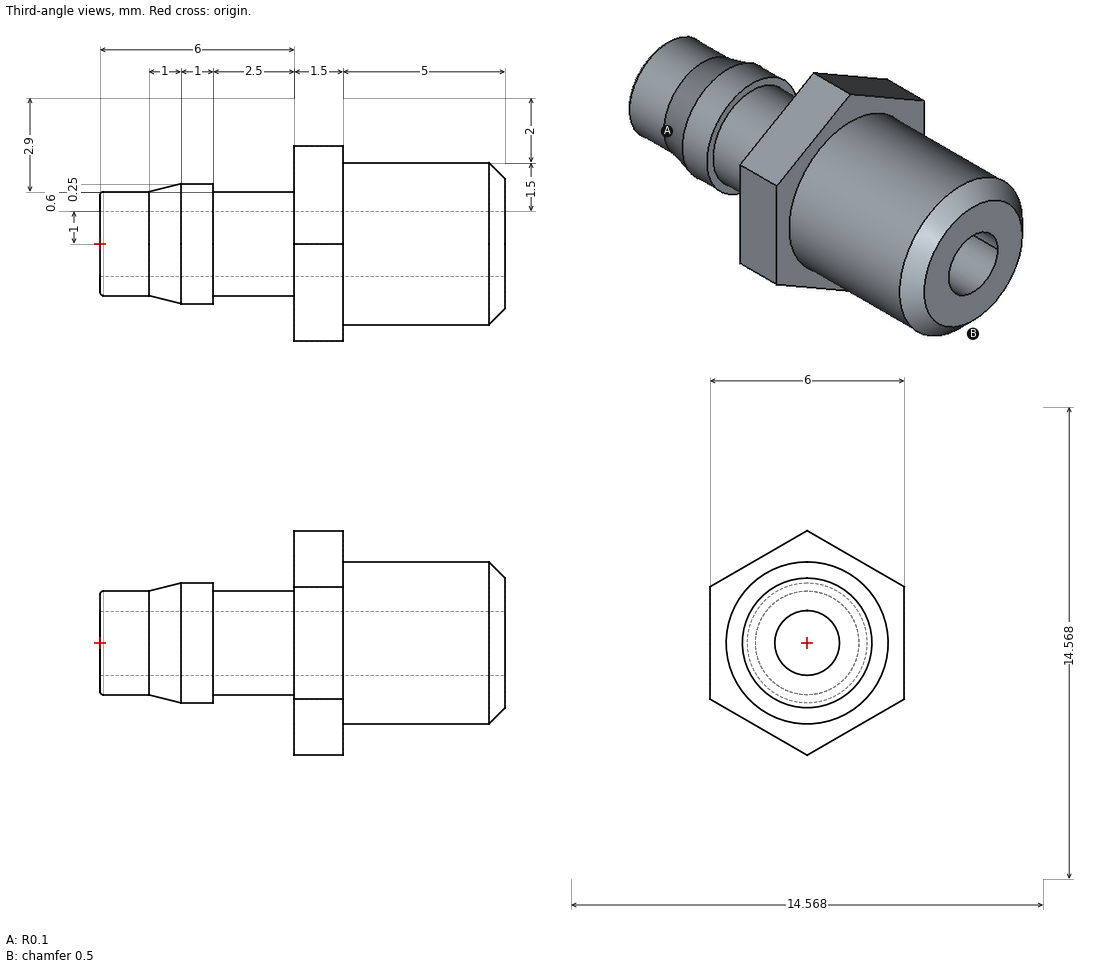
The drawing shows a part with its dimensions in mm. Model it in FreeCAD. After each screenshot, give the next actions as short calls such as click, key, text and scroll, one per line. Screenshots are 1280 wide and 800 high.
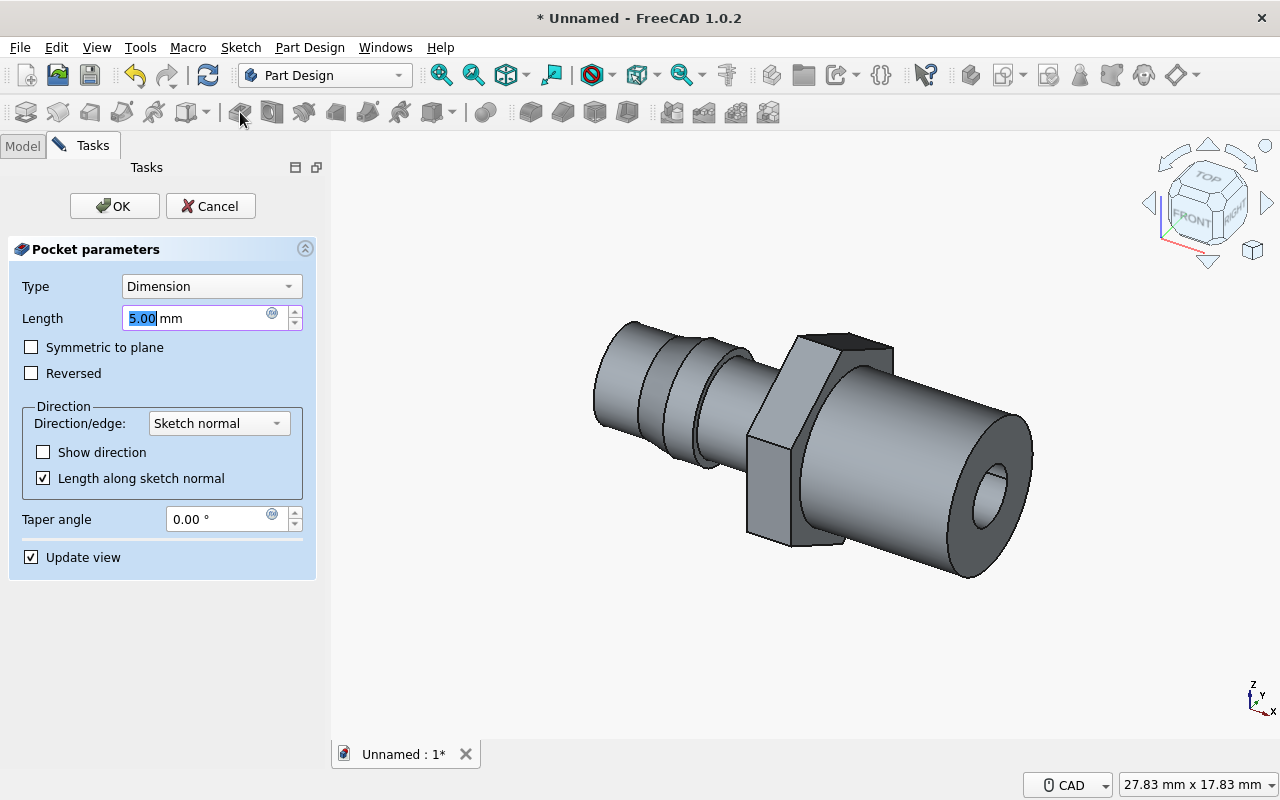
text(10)
key(Tab)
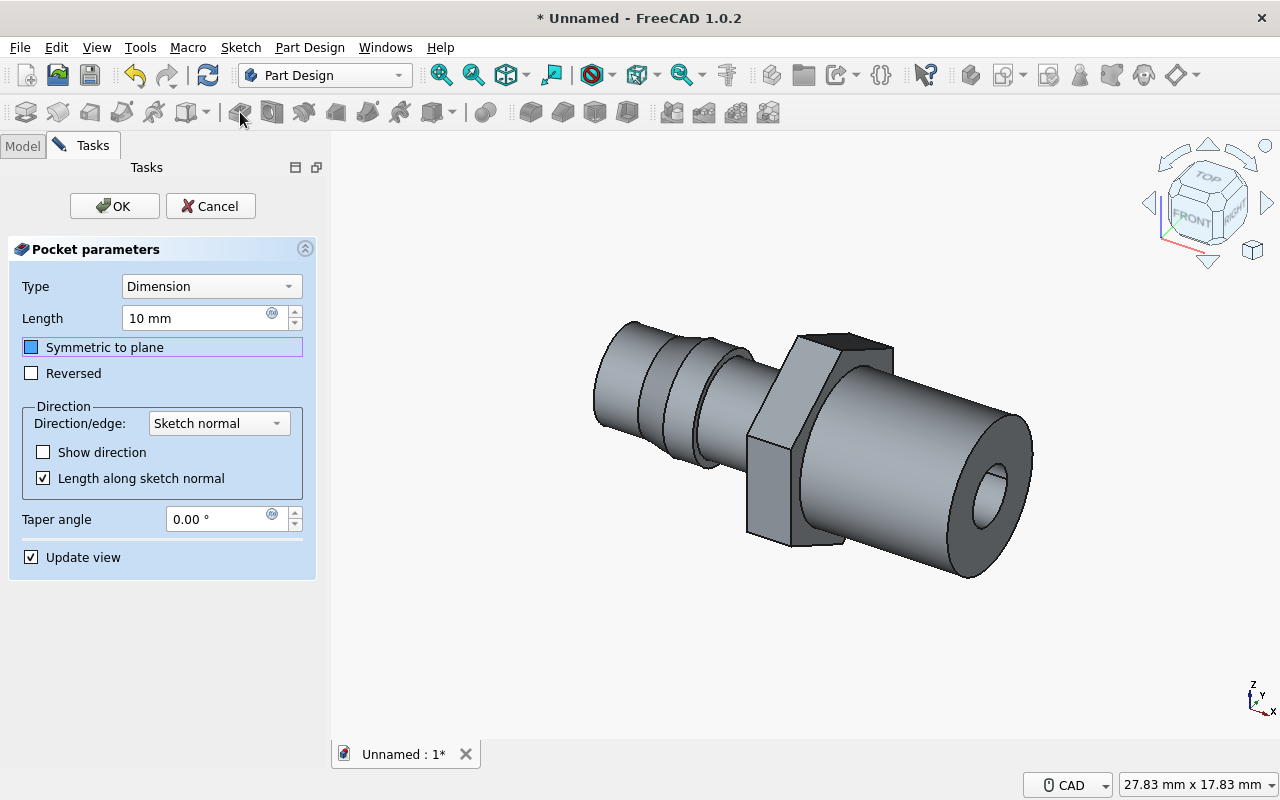
click(115, 206)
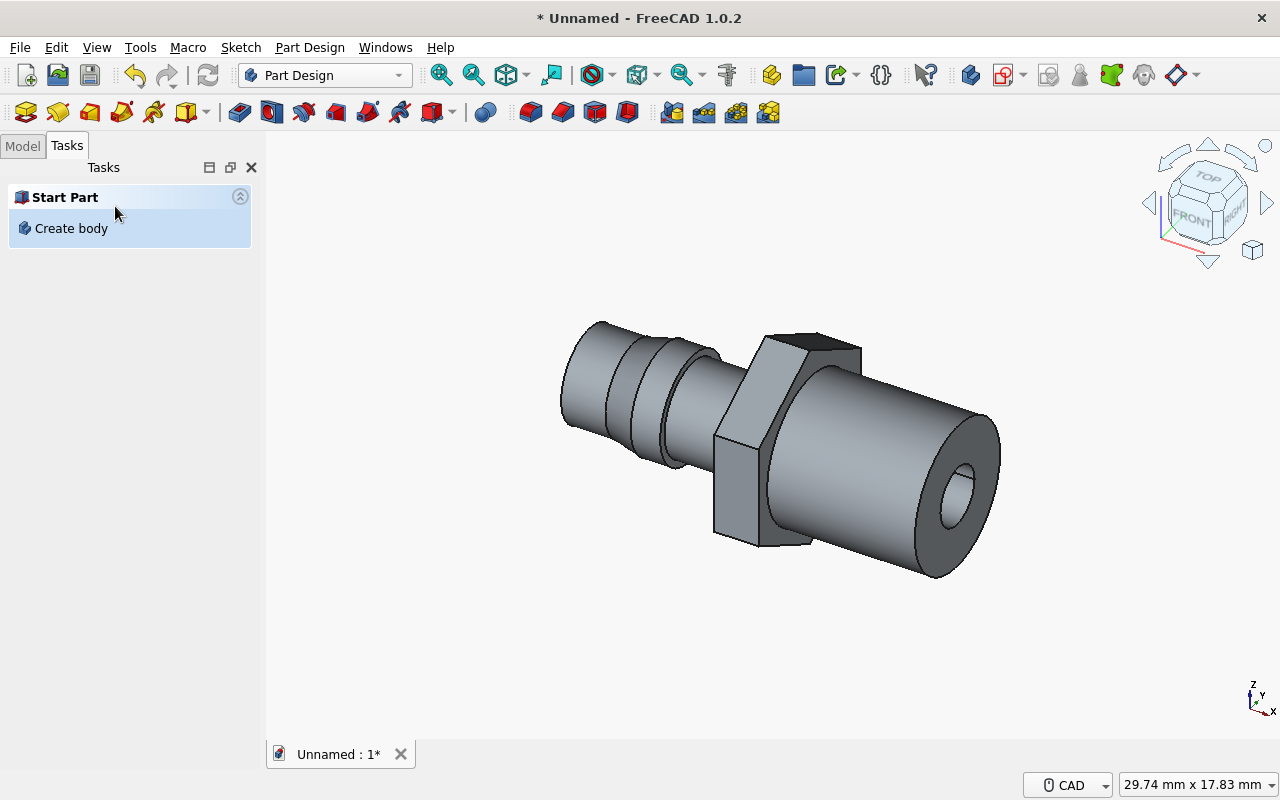
click(566, 421)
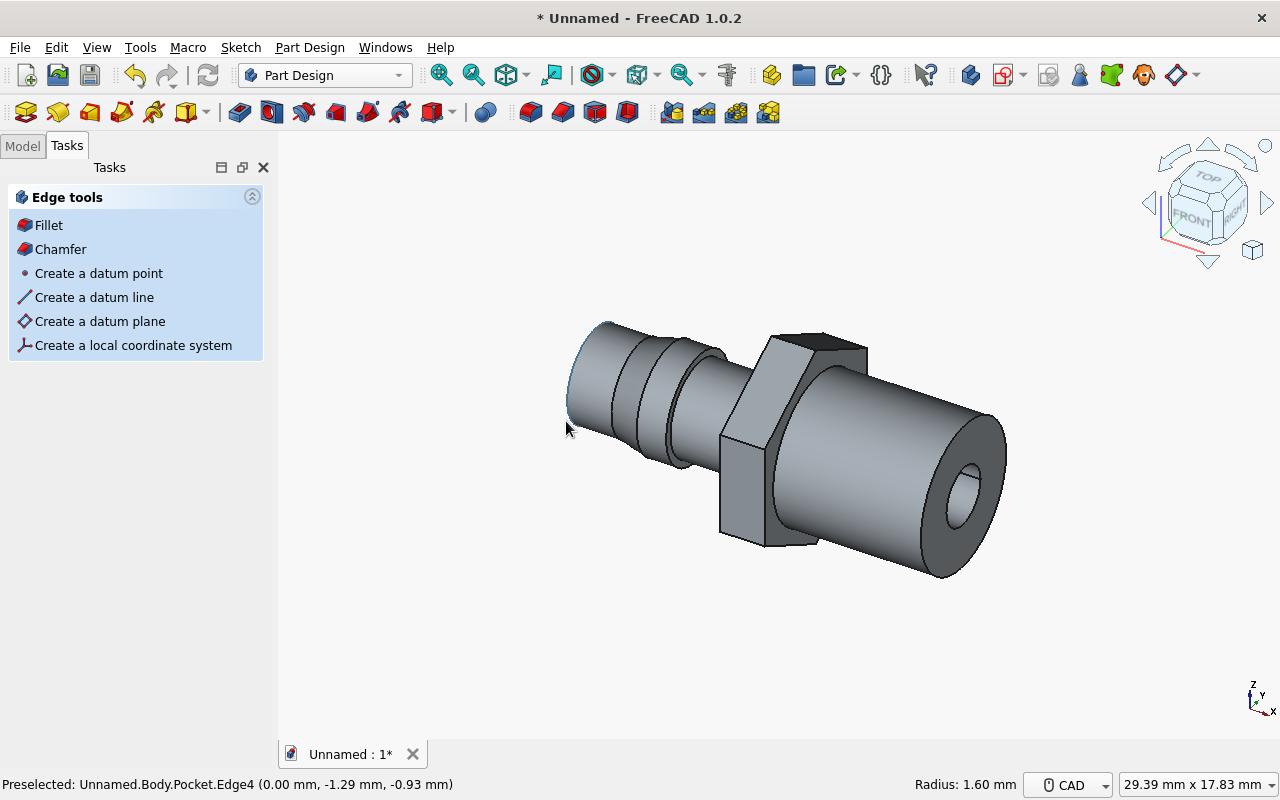
click(532, 112)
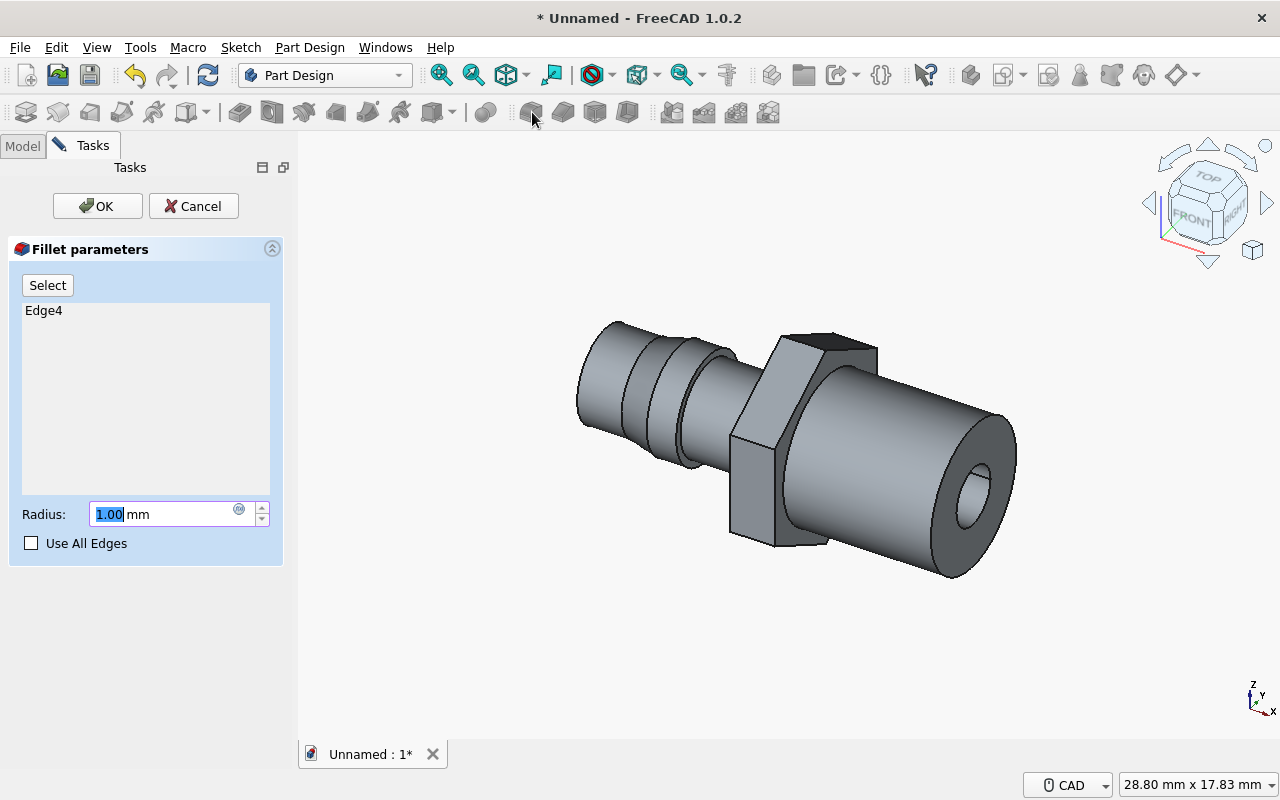
text(0.1)
key(Tab)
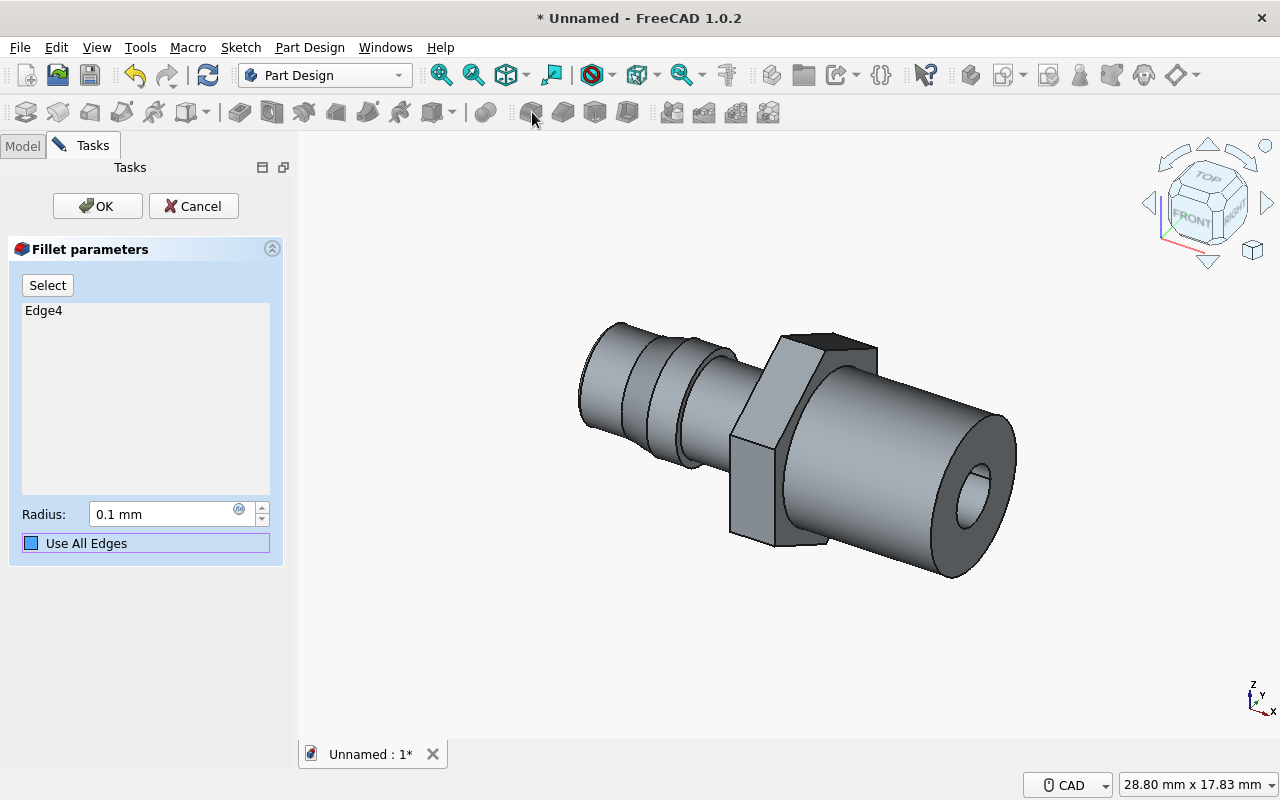
click(98, 206)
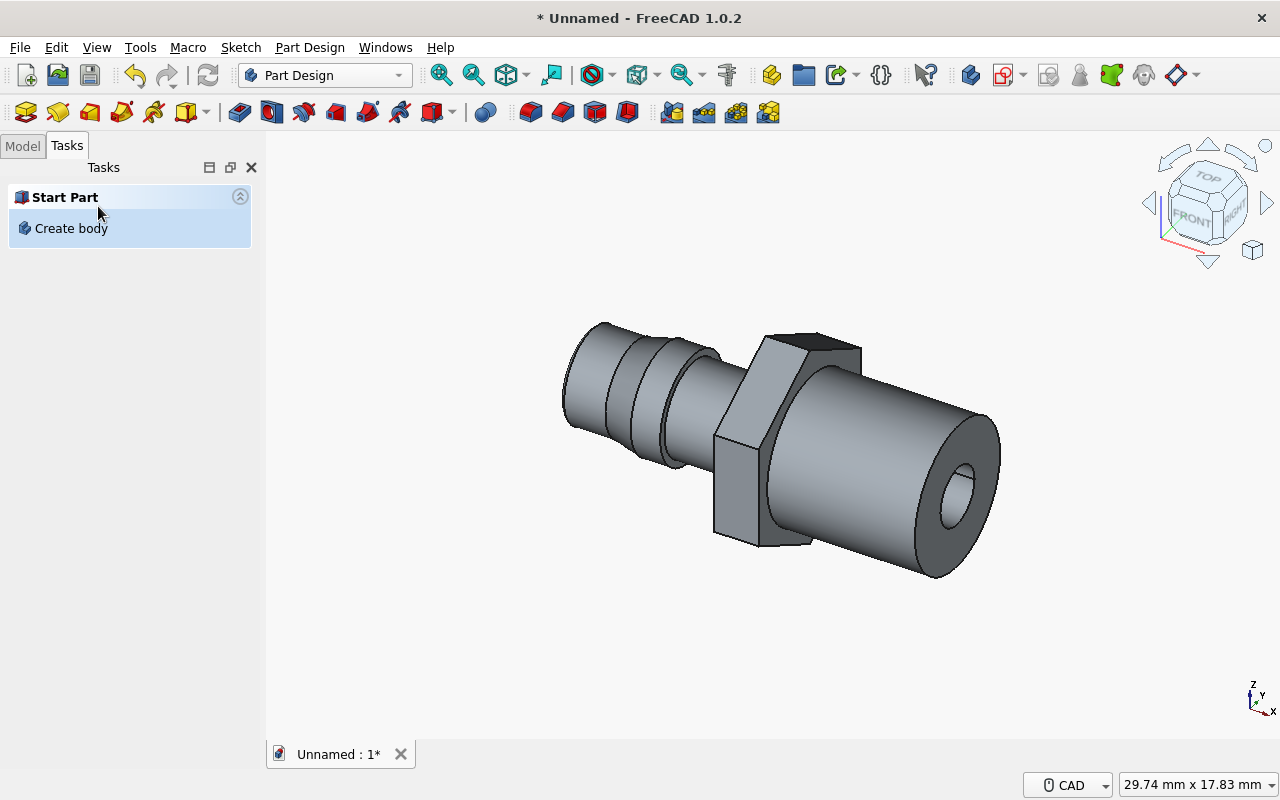
click(915, 538)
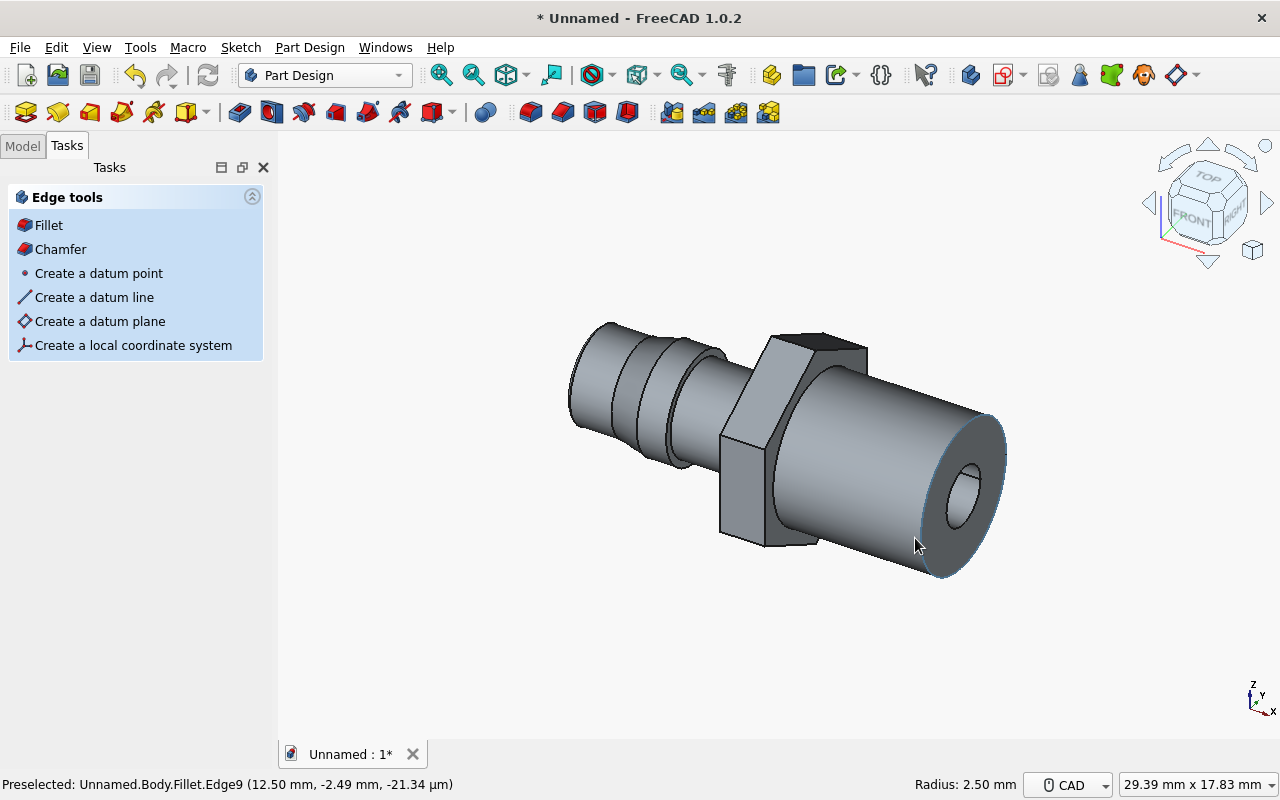
click(564, 112)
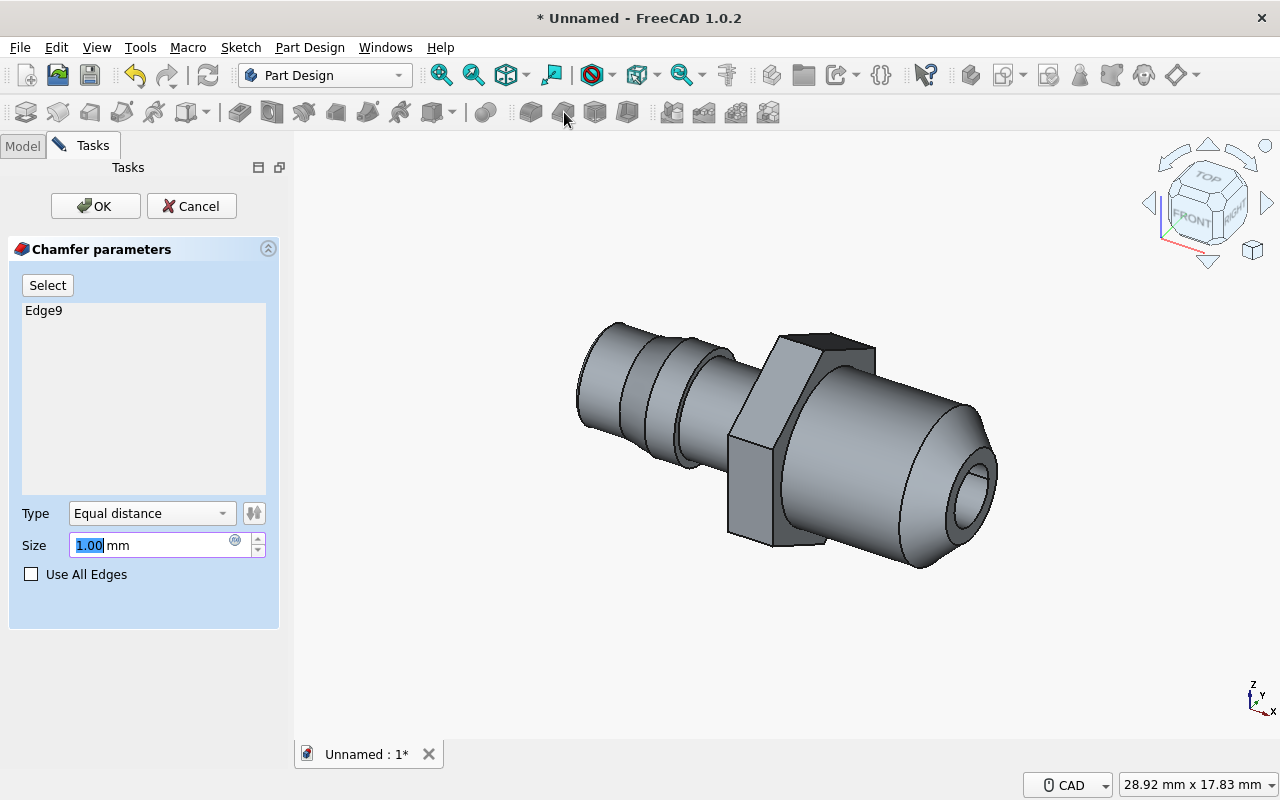
text(0.5)
key(Tab)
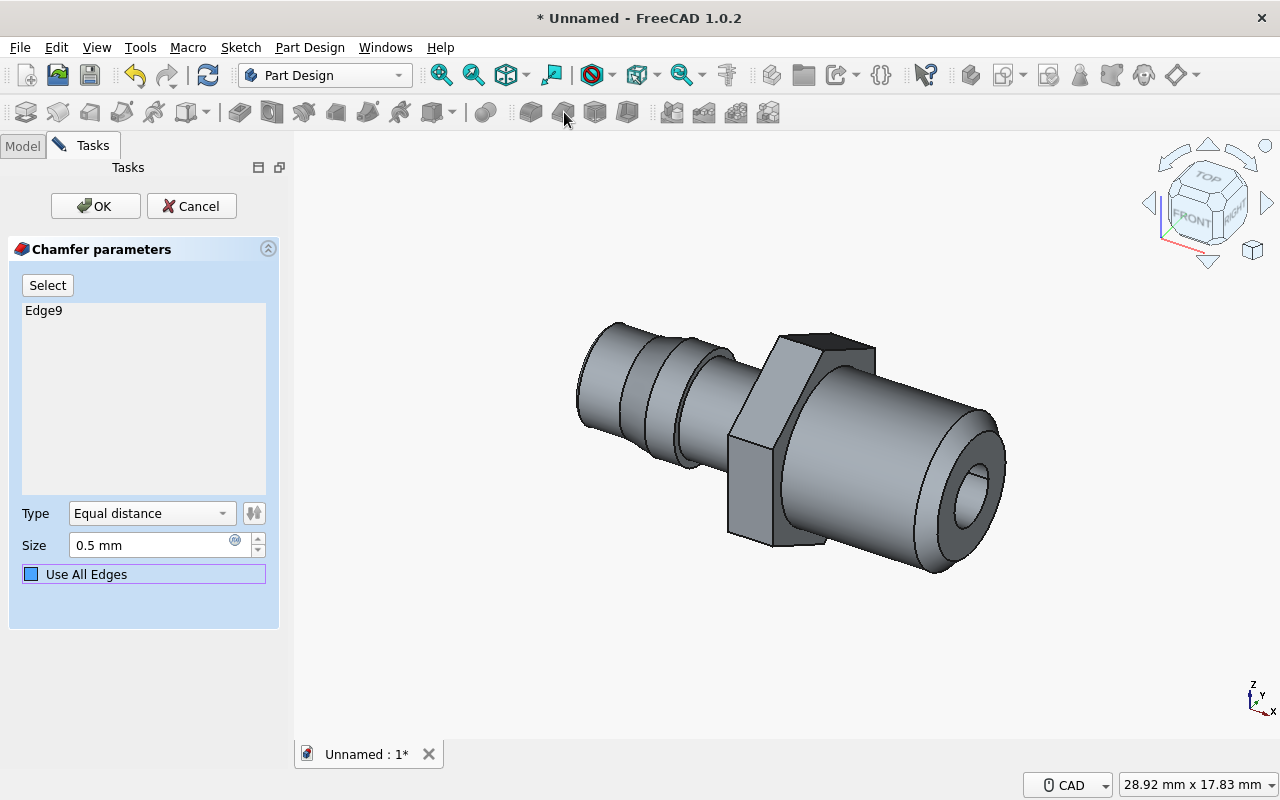
click(96, 206)